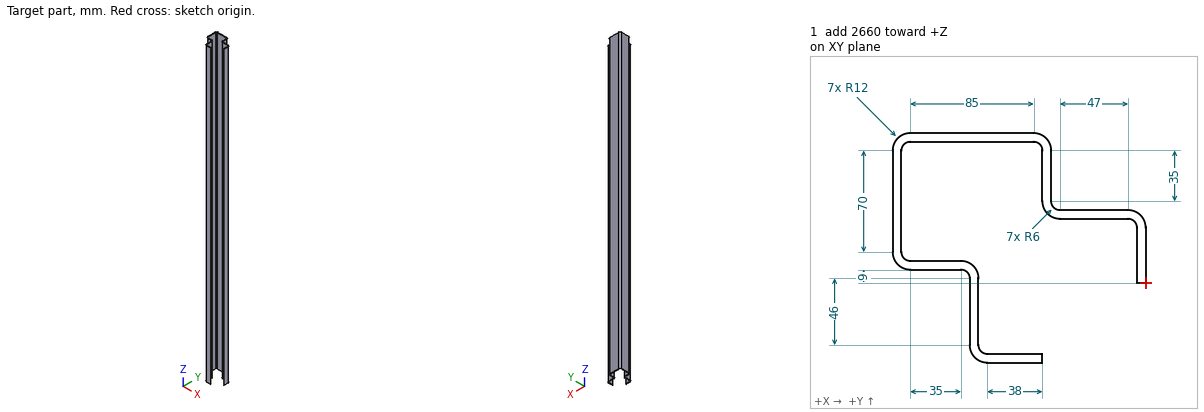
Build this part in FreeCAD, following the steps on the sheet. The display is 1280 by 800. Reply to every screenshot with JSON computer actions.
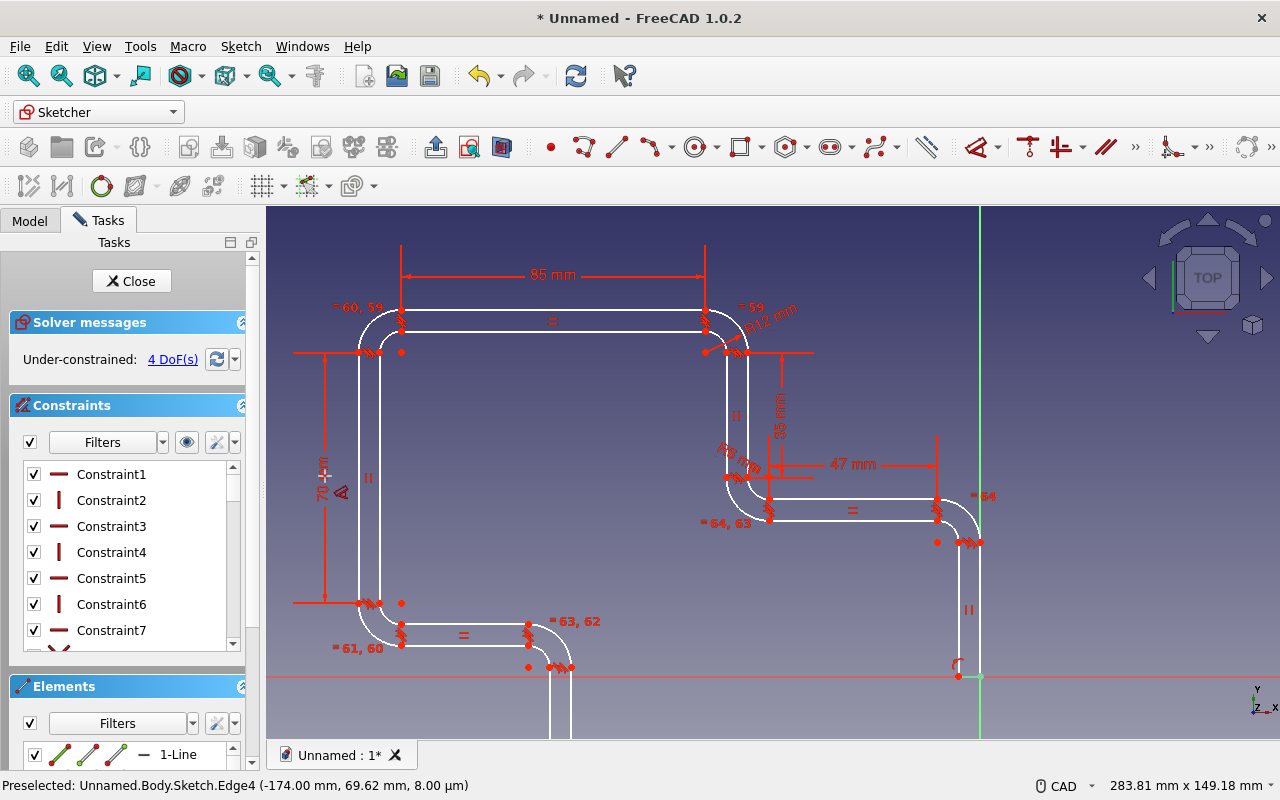
{"action": "left_click", "coordinate": [439, 646]}
{"action": "left_click", "coordinate": [465, 704]}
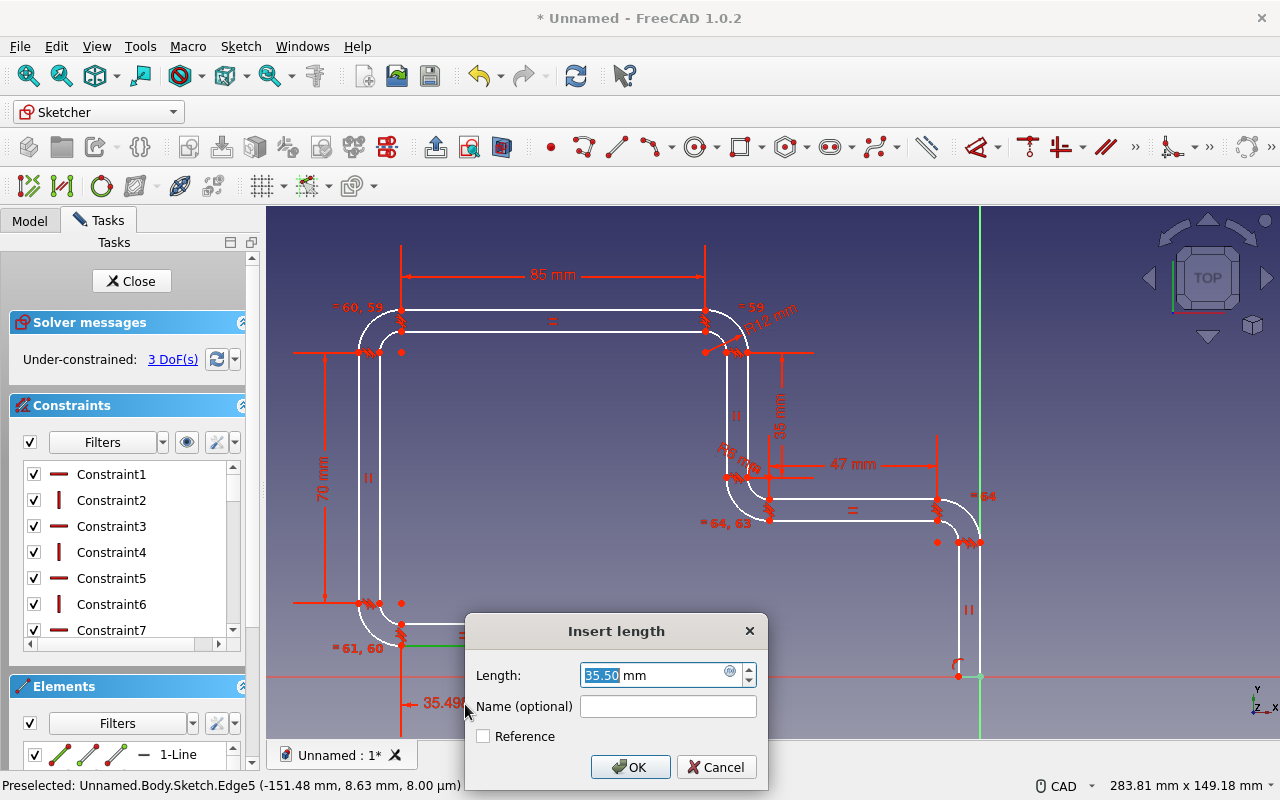
{"action": "type", "text": "35"}
{"action": "key", "text": "Return"}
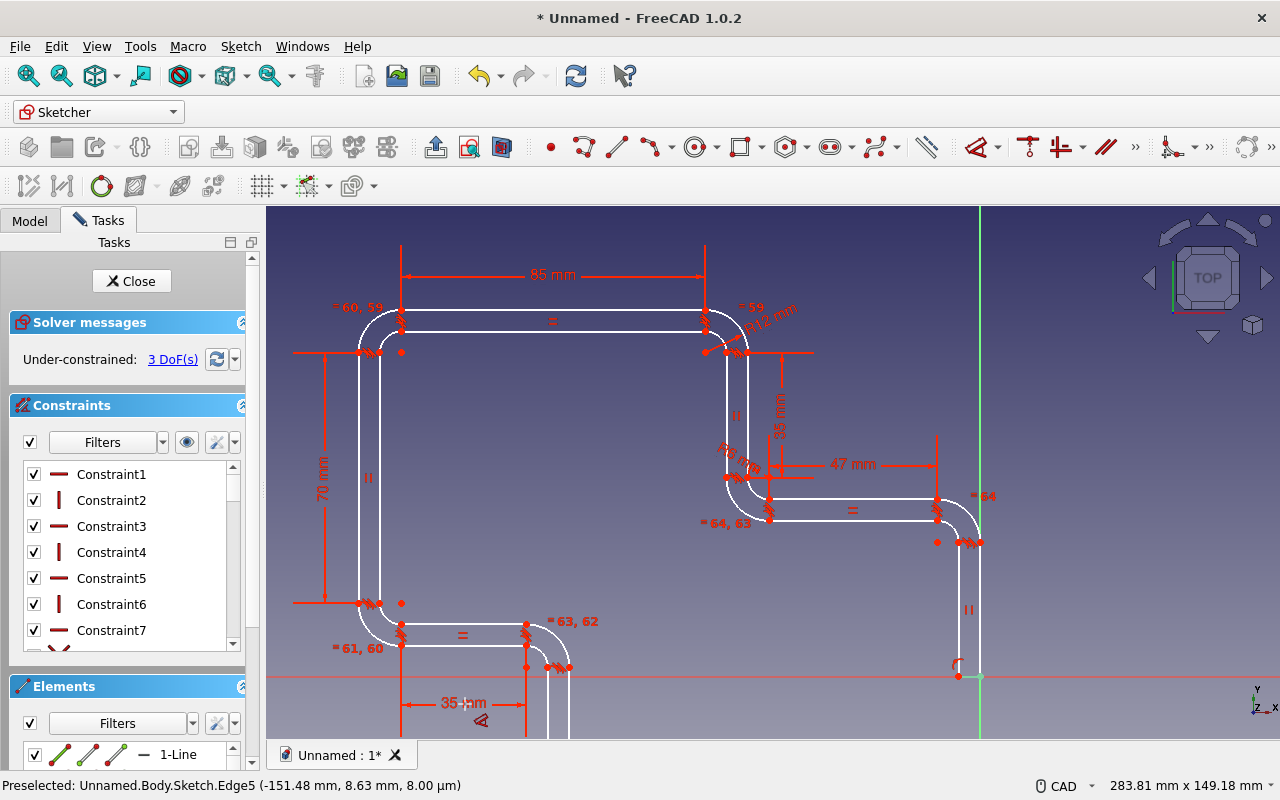
{"action": "left_click", "coordinate": [548, 699]}
{"action": "left_click", "coordinate": [606, 699]}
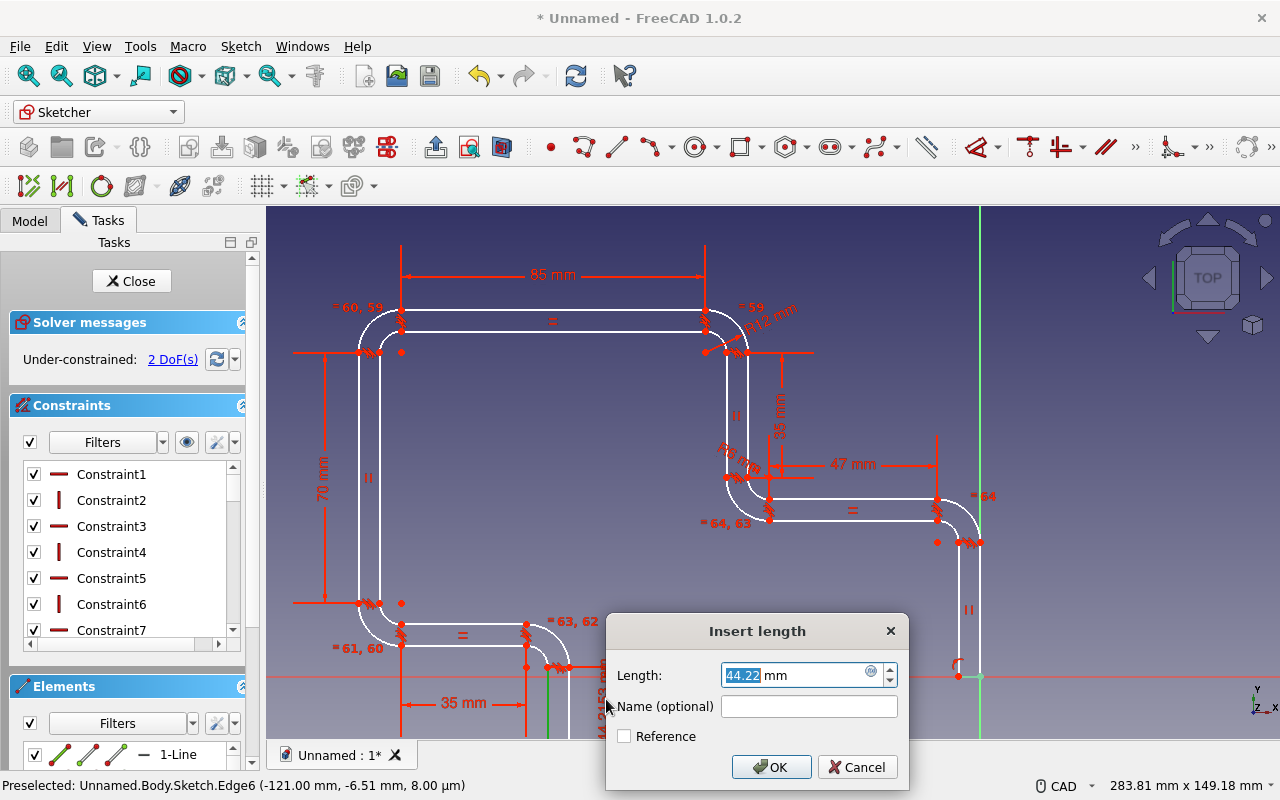
{"action": "type", "text": "46"}
{"action": "key", "text": "Return"}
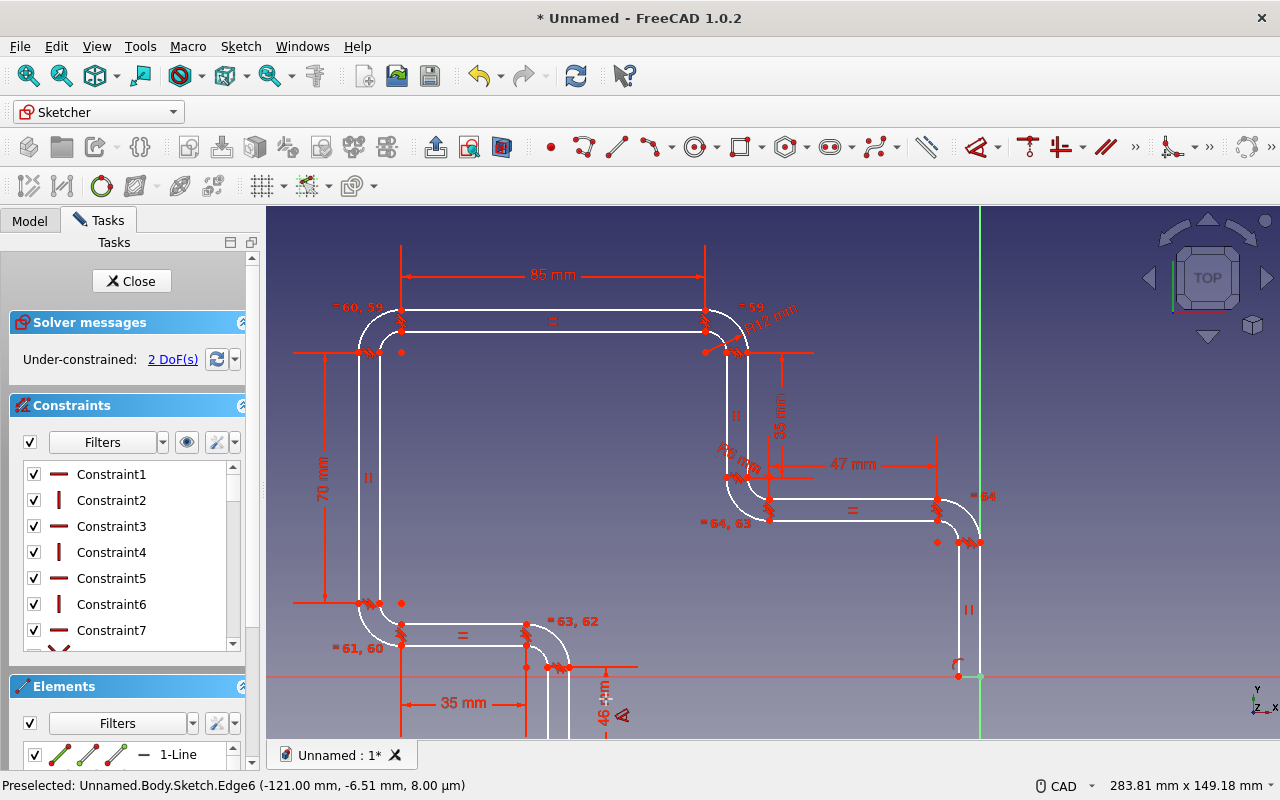
{"action": "scroll", "coordinate": [747, 328], "scroll_direction": "down", "scroll_amount": 3}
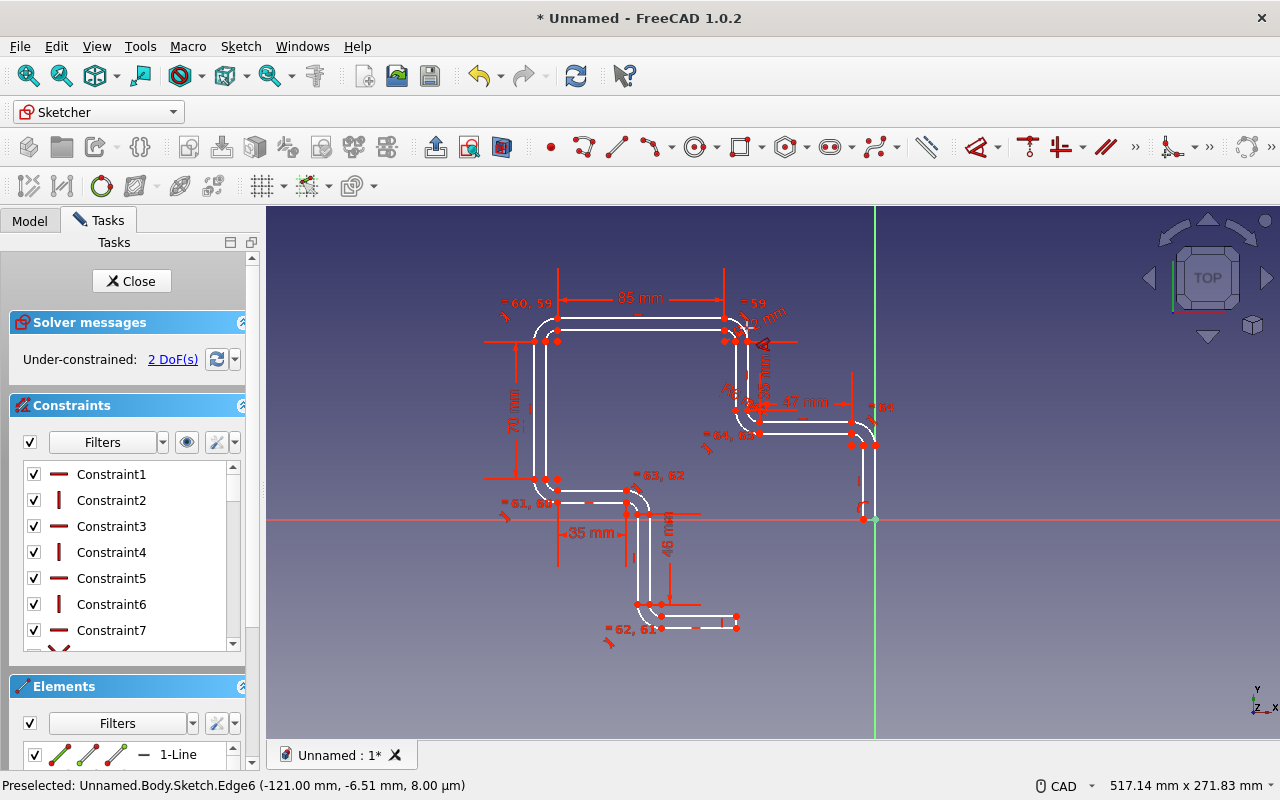
{"action": "left_click", "coordinate": [684, 628]}
{"action": "left_click", "coordinate": [699, 662]}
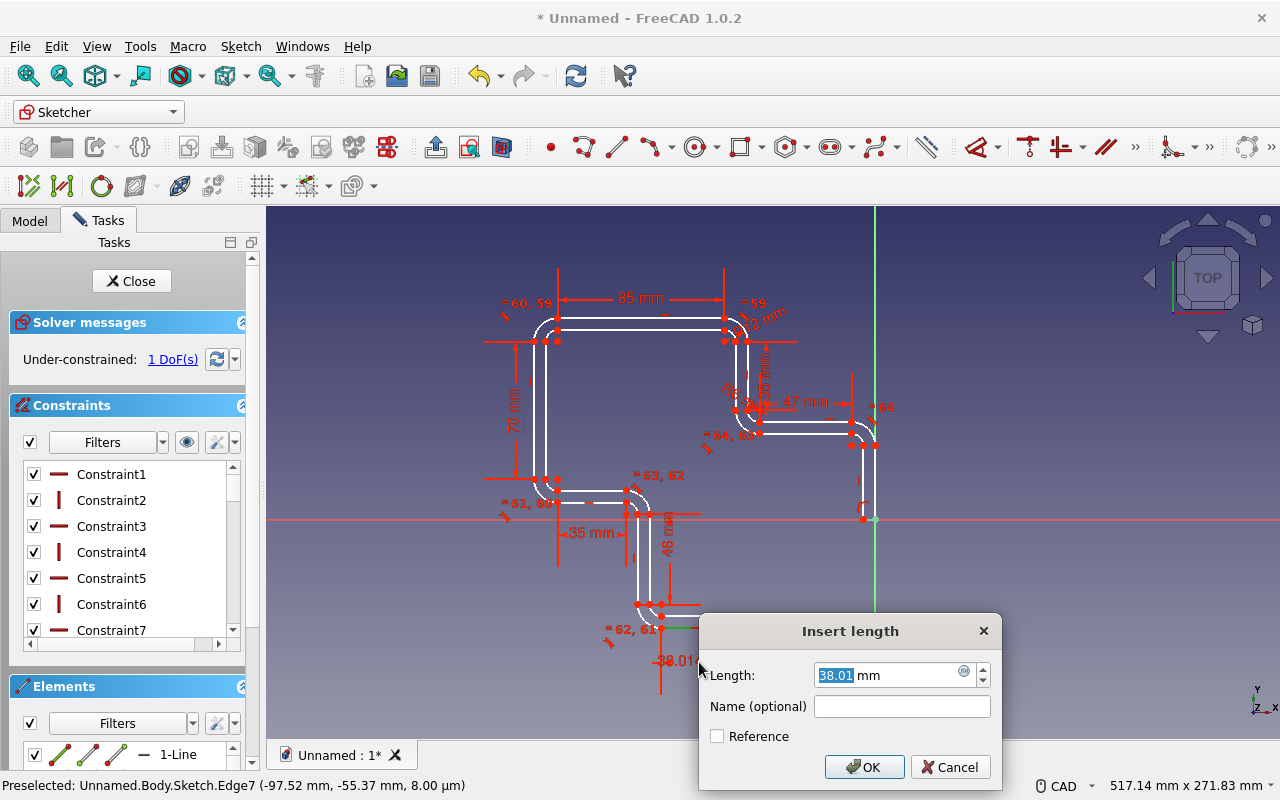
{"action": "type", "text": "38"}
{"action": "key", "text": "Return"}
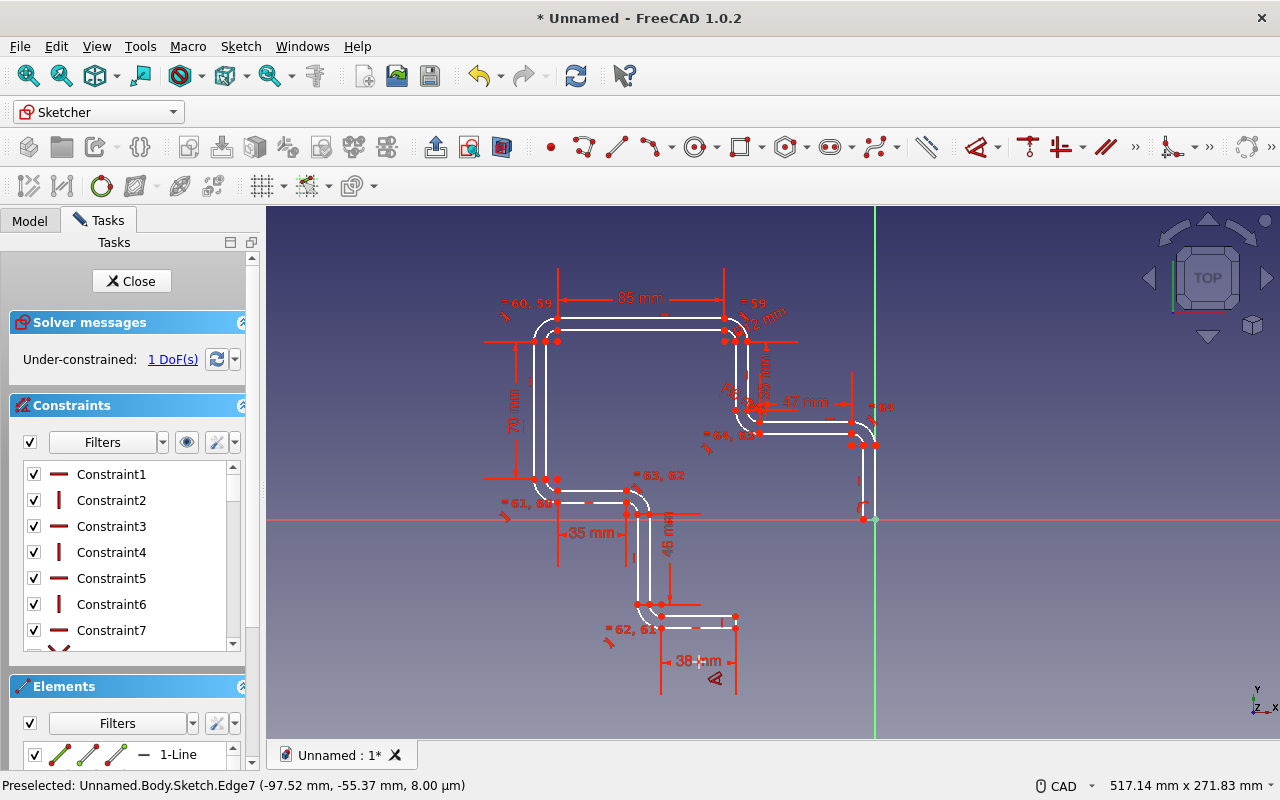
{"action": "scroll", "coordinate": [558, 503], "scroll_direction": "up", "scroll_amount": 5}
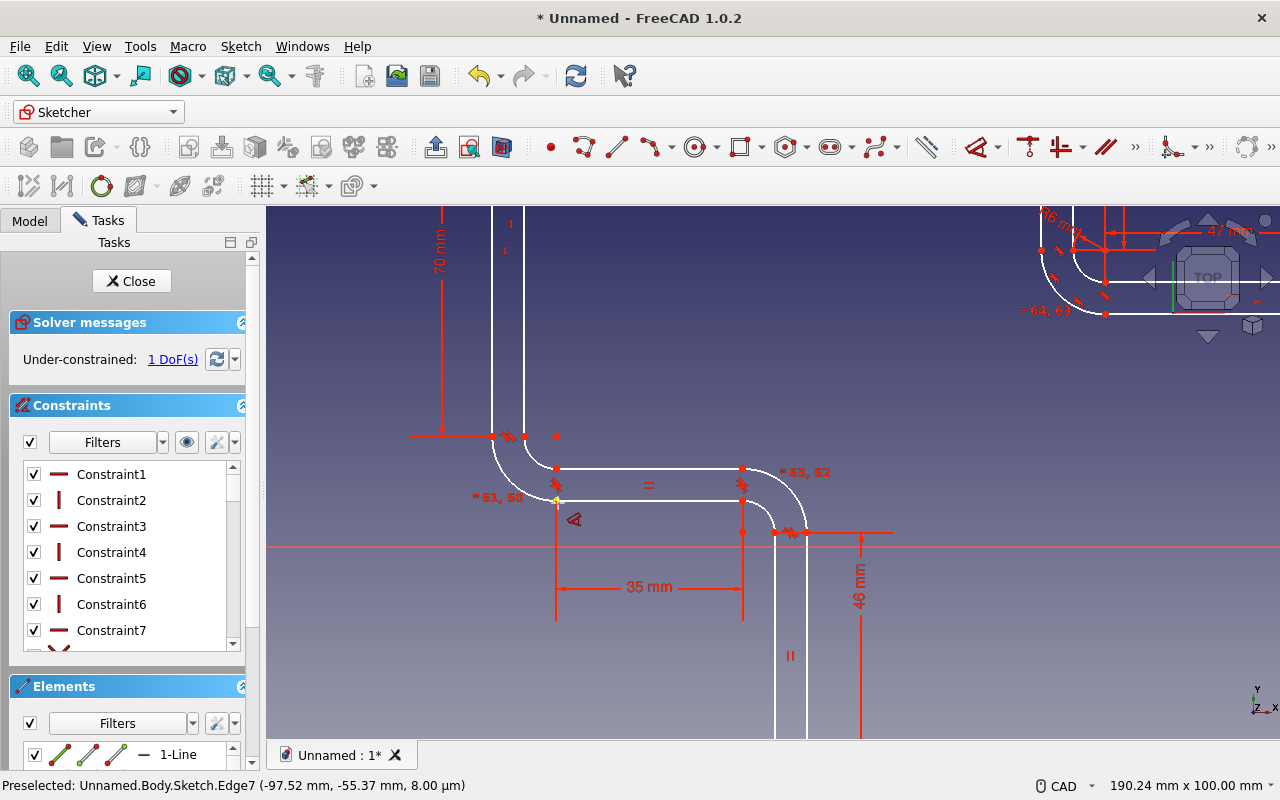
{"action": "left_click", "coordinate": [556, 501]}
{"action": "left_click", "coordinate": [522, 524]}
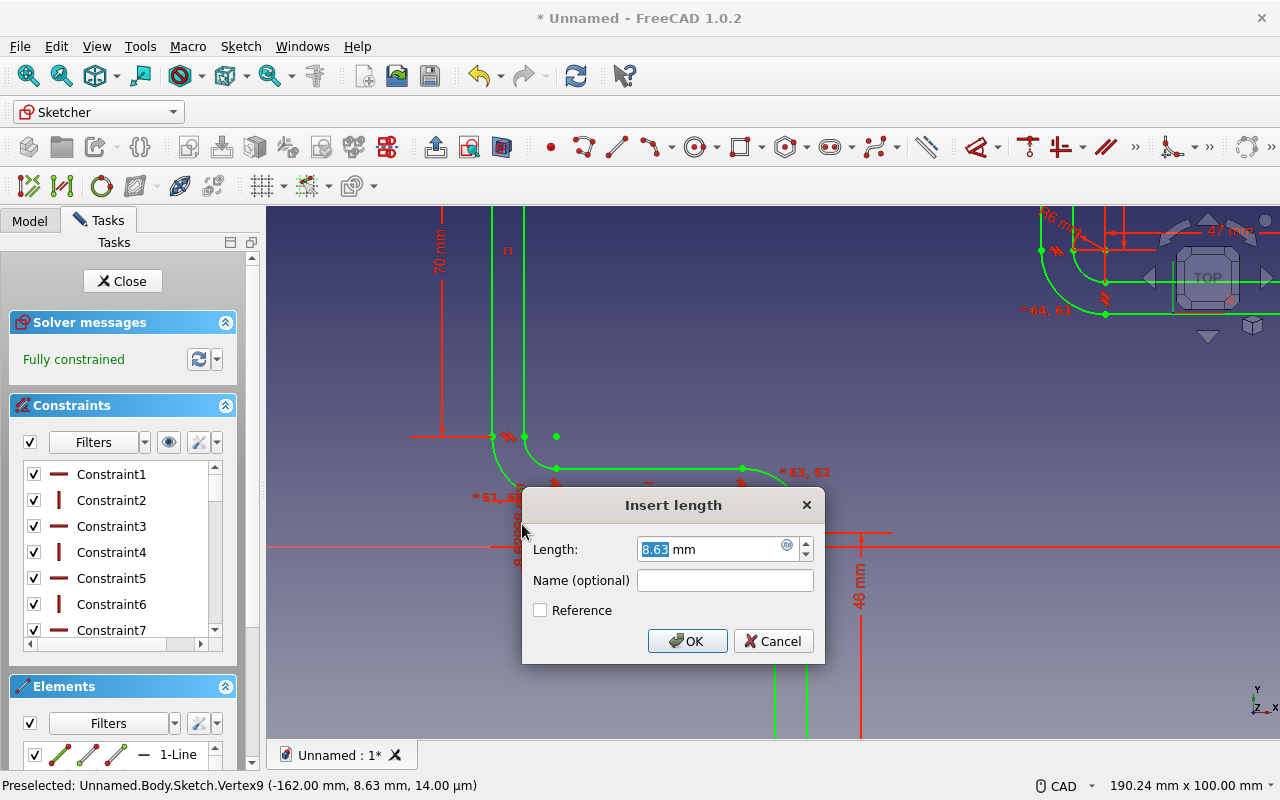
{"action": "type", "text": "9"}
{"action": "key", "text": "Return"}
{"action": "key", "text": "Escape"}